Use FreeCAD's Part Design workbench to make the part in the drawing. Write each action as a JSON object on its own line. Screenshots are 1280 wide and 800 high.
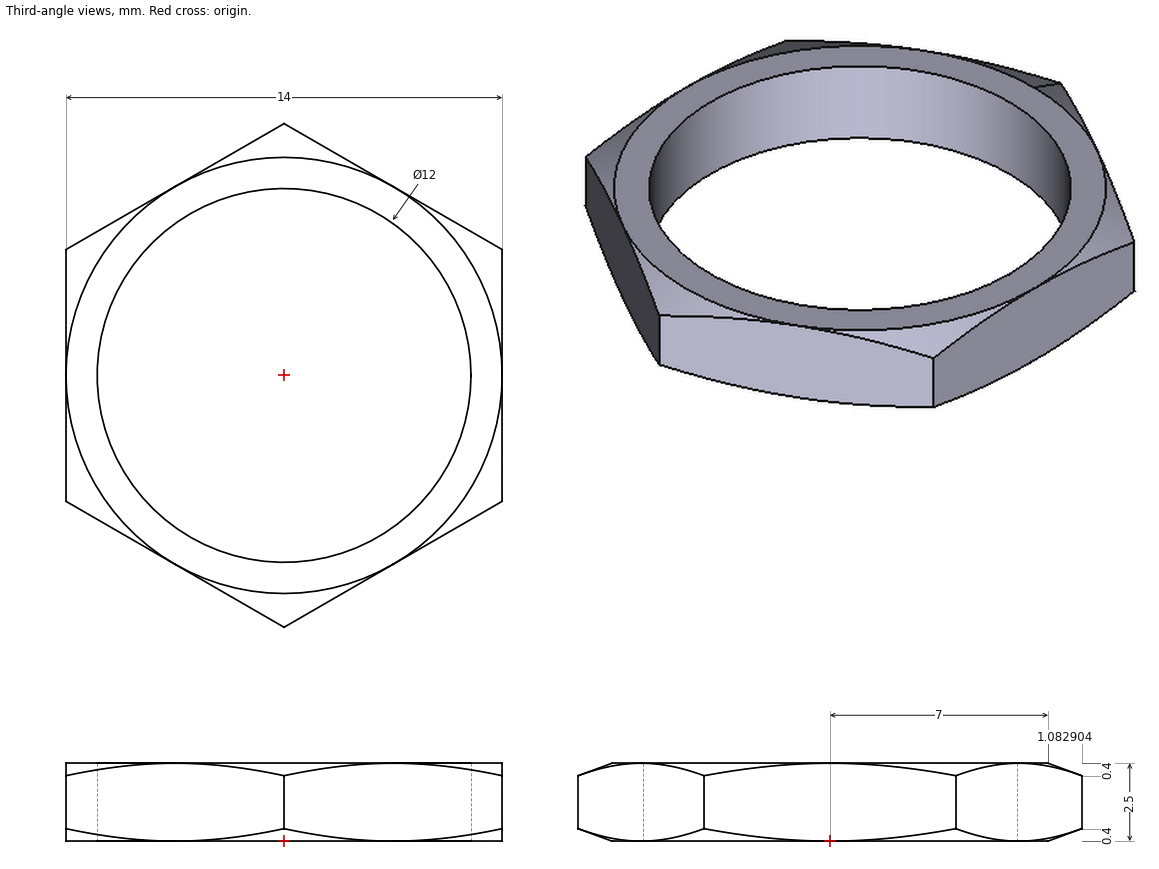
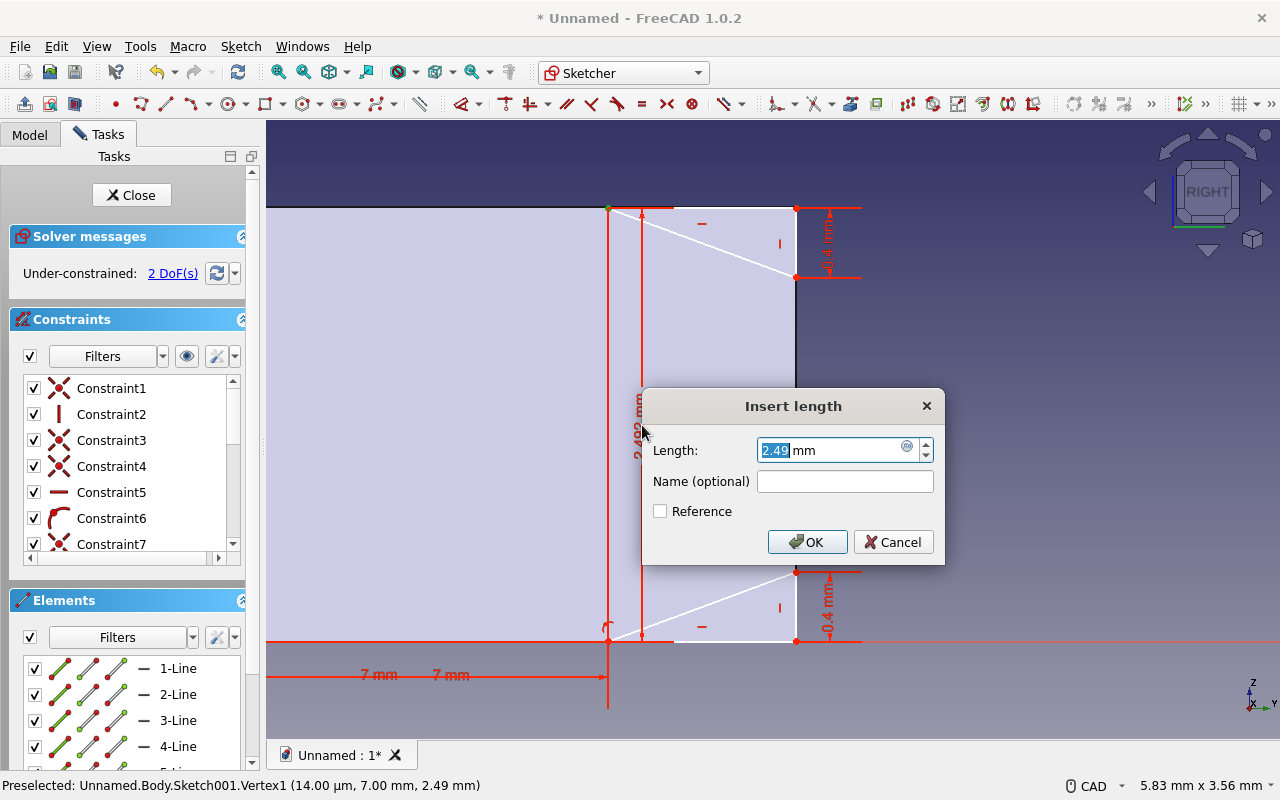
{"action": "type", "text": "2.5"}
{"action": "key", "text": "Return"}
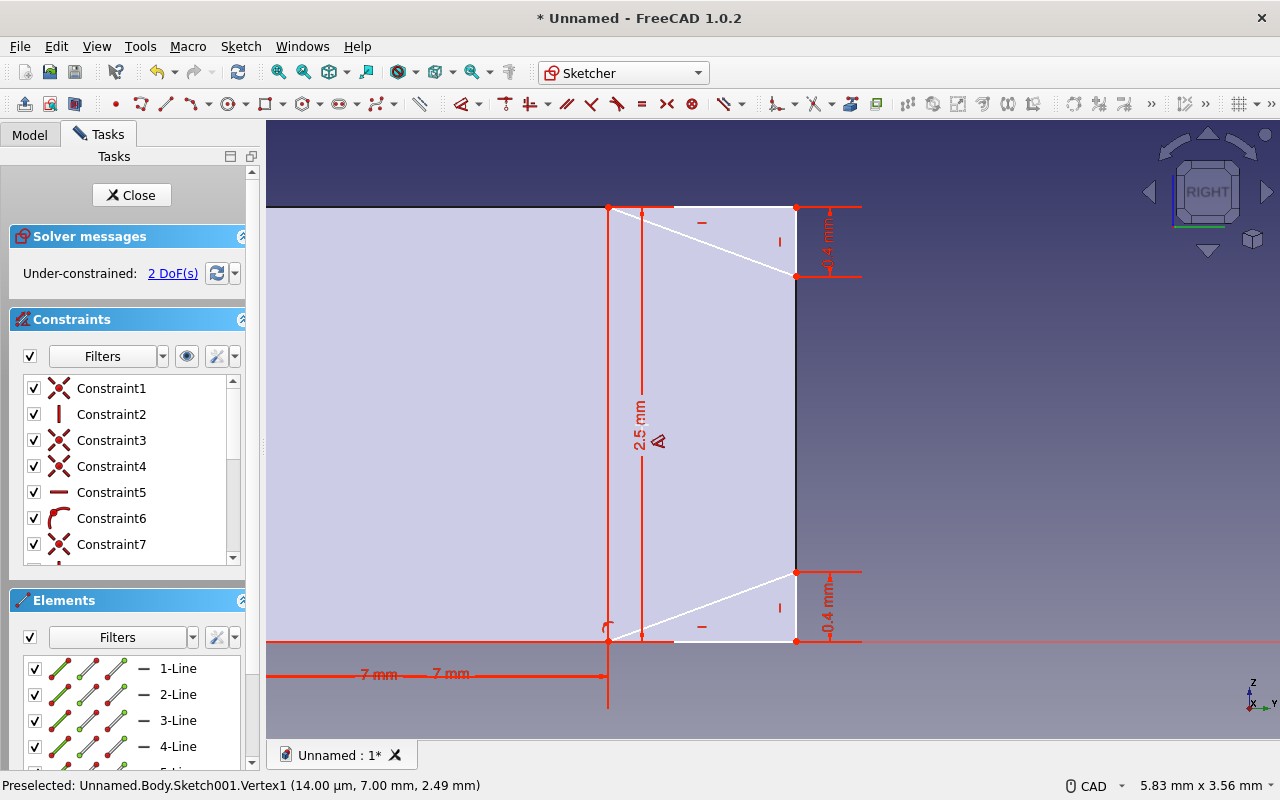
{"action": "left_click", "coordinate": [740, 207]}
{"action": "left_click", "coordinate": [702, 173]}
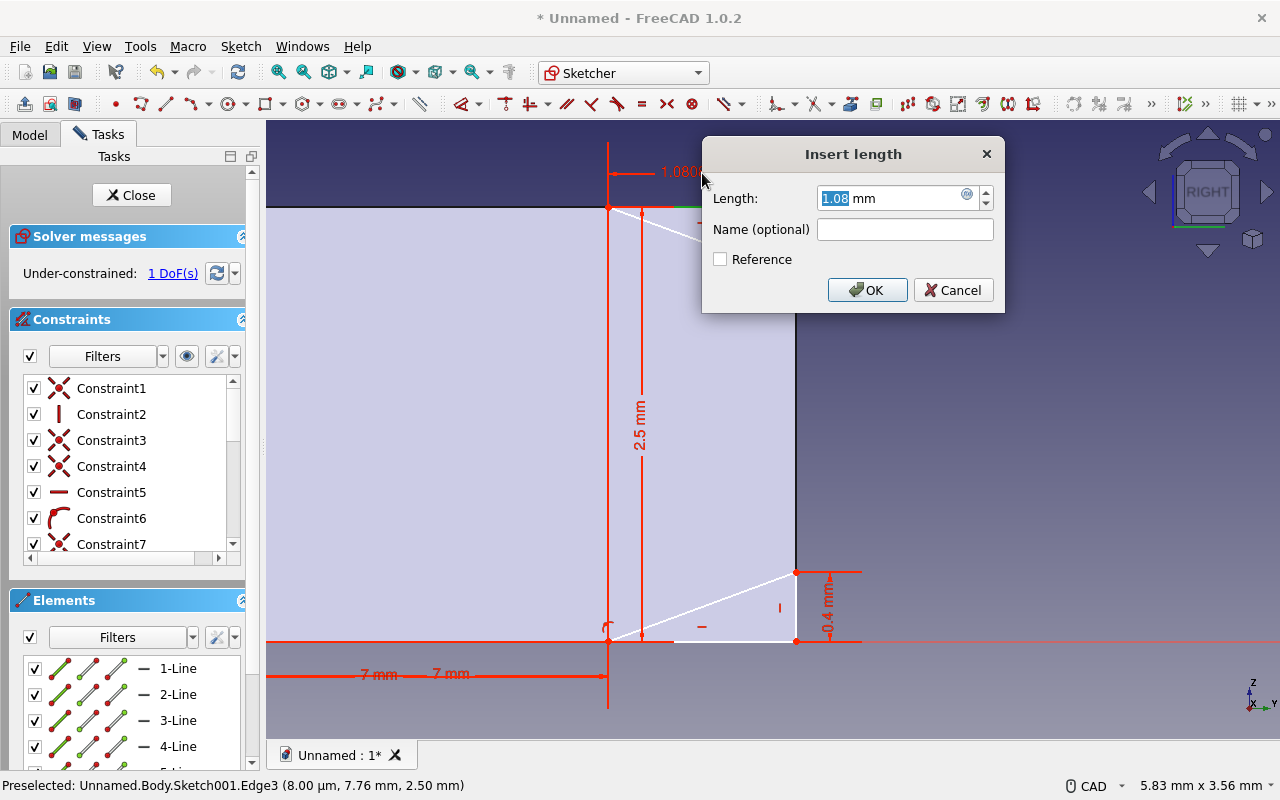
{"action": "type", "text": "1.082904"}
{"action": "key", "text": "Return"}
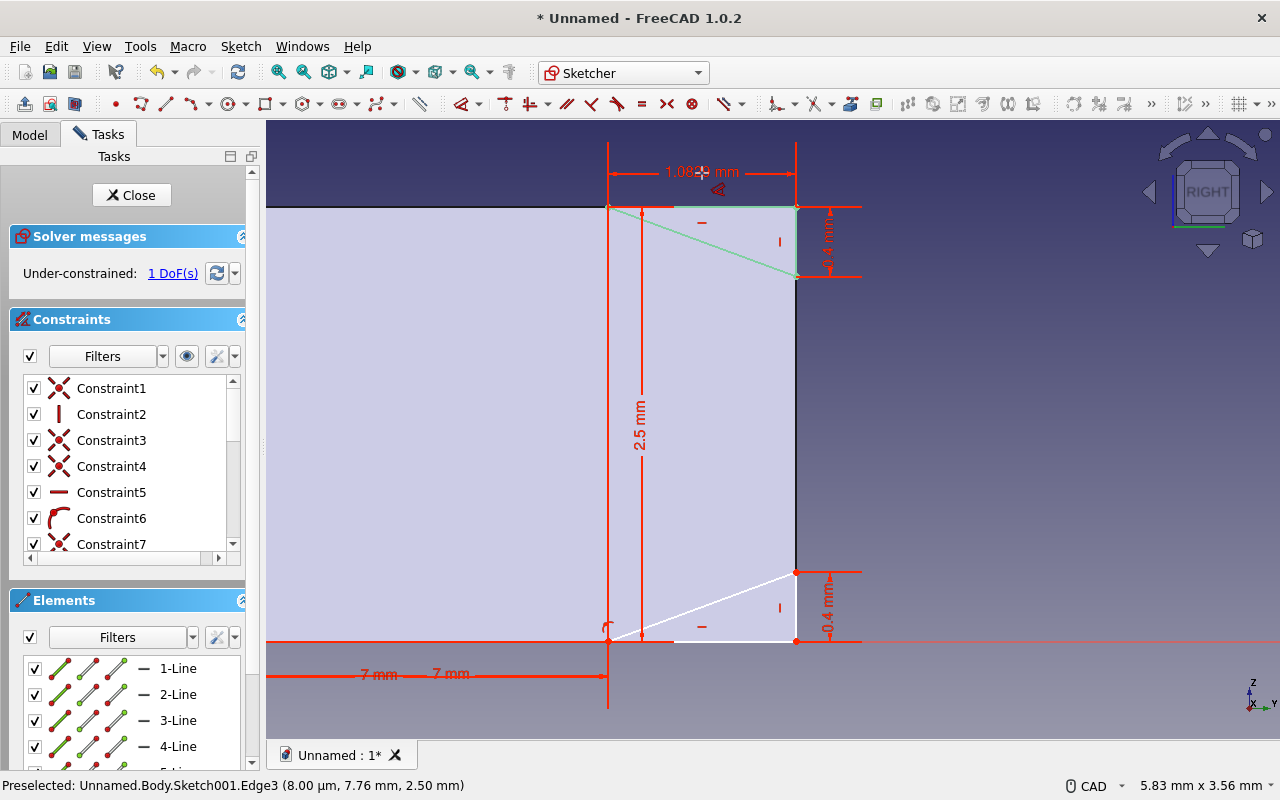
{"action": "left_click", "coordinate": [664, 642]}
{"action": "left_click", "coordinate": [702, 676]}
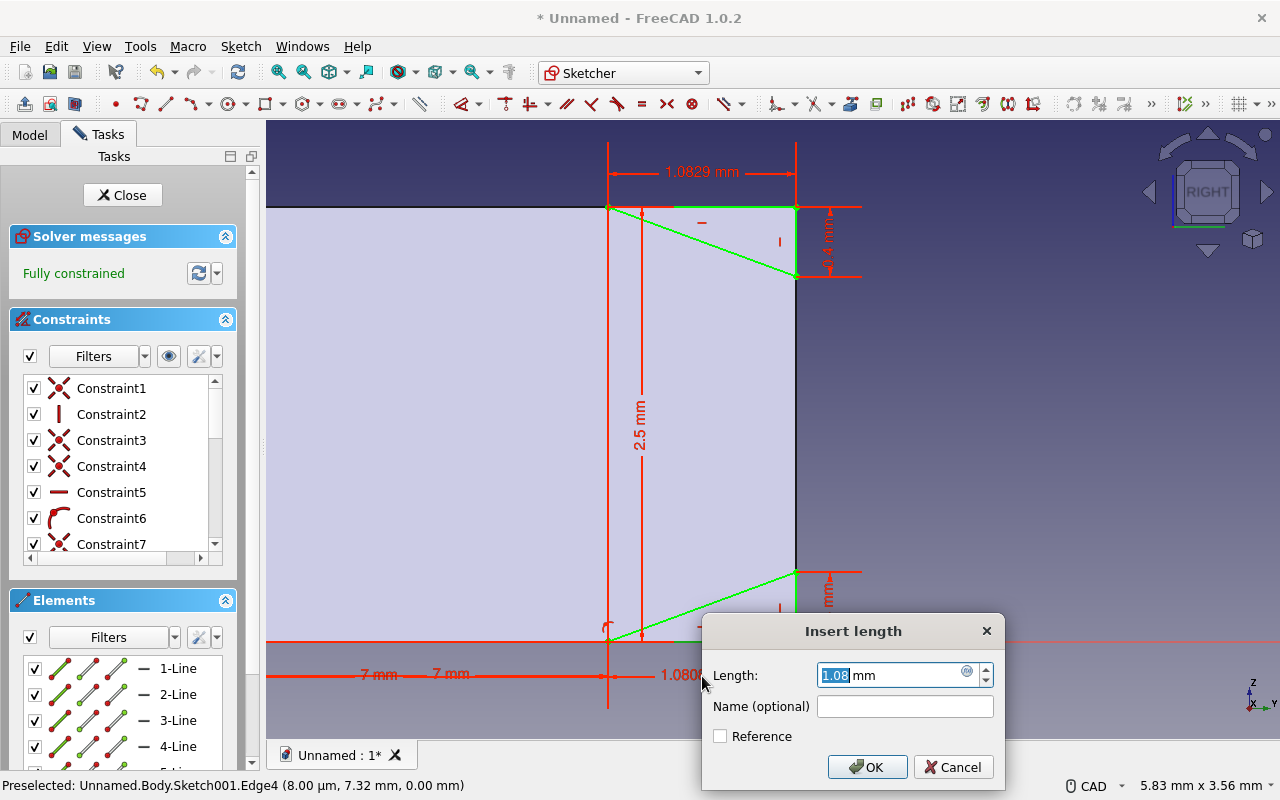
{"action": "type", "text": "1.082904"}
{"action": "key", "text": "Return"}
{"action": "key", "text": "Escape"}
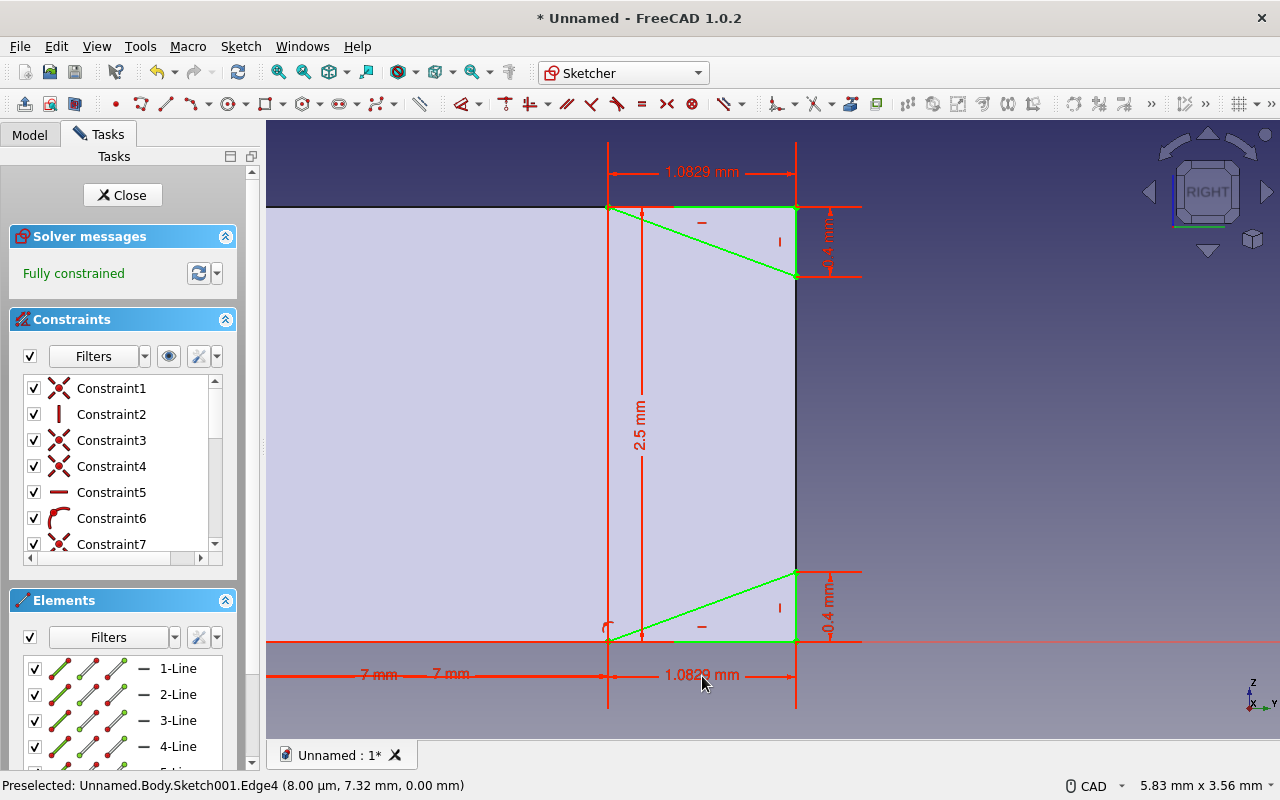
{"action": "left_click", "coordinate": [123, 195]}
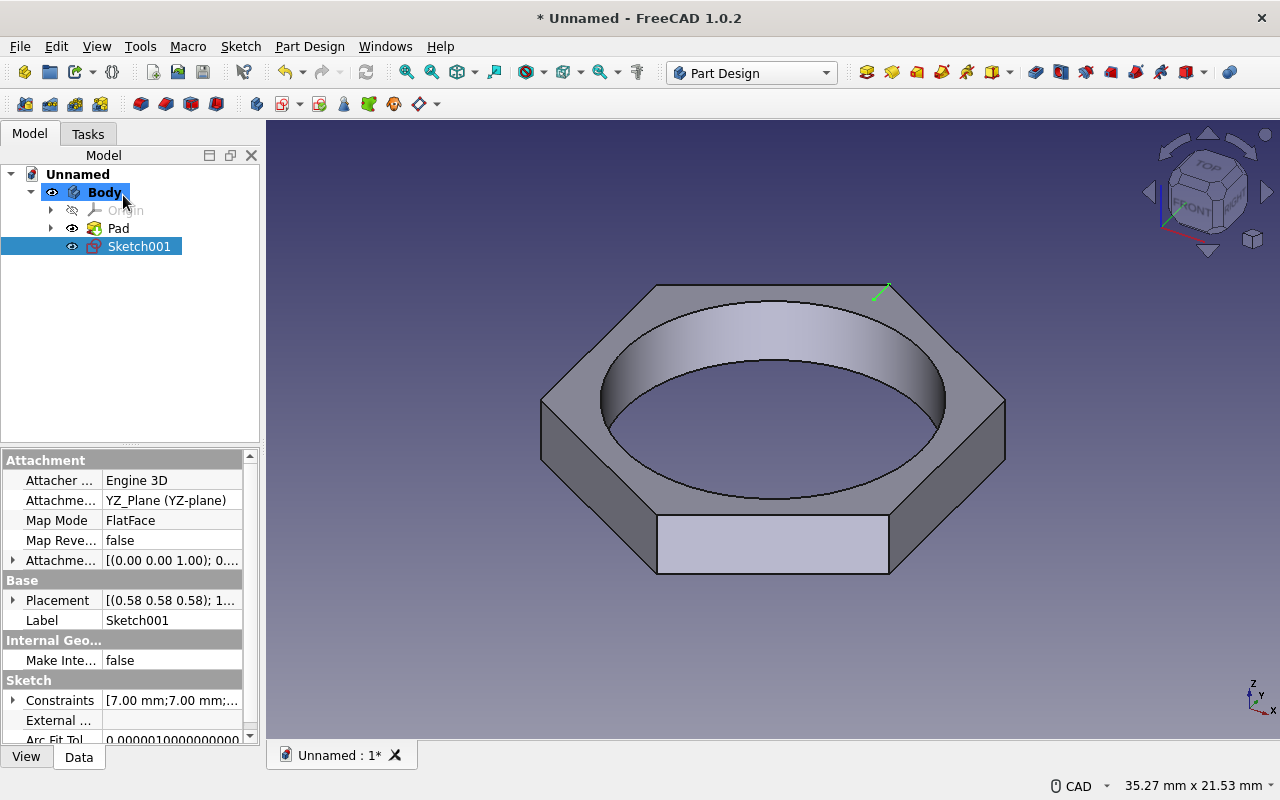
{"action": "left_click", "coordinate": [1086, 72]}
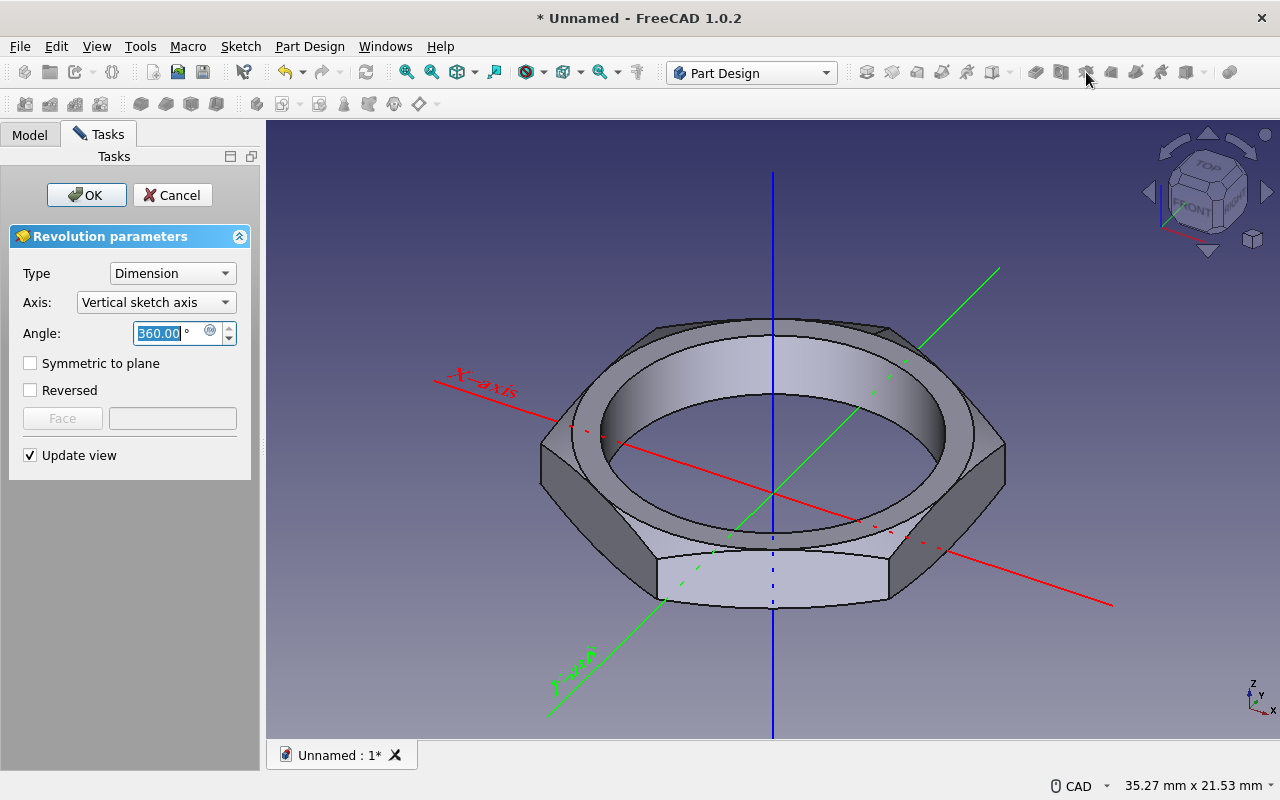
{"action": "left_click", "coordinate": [87, 195]}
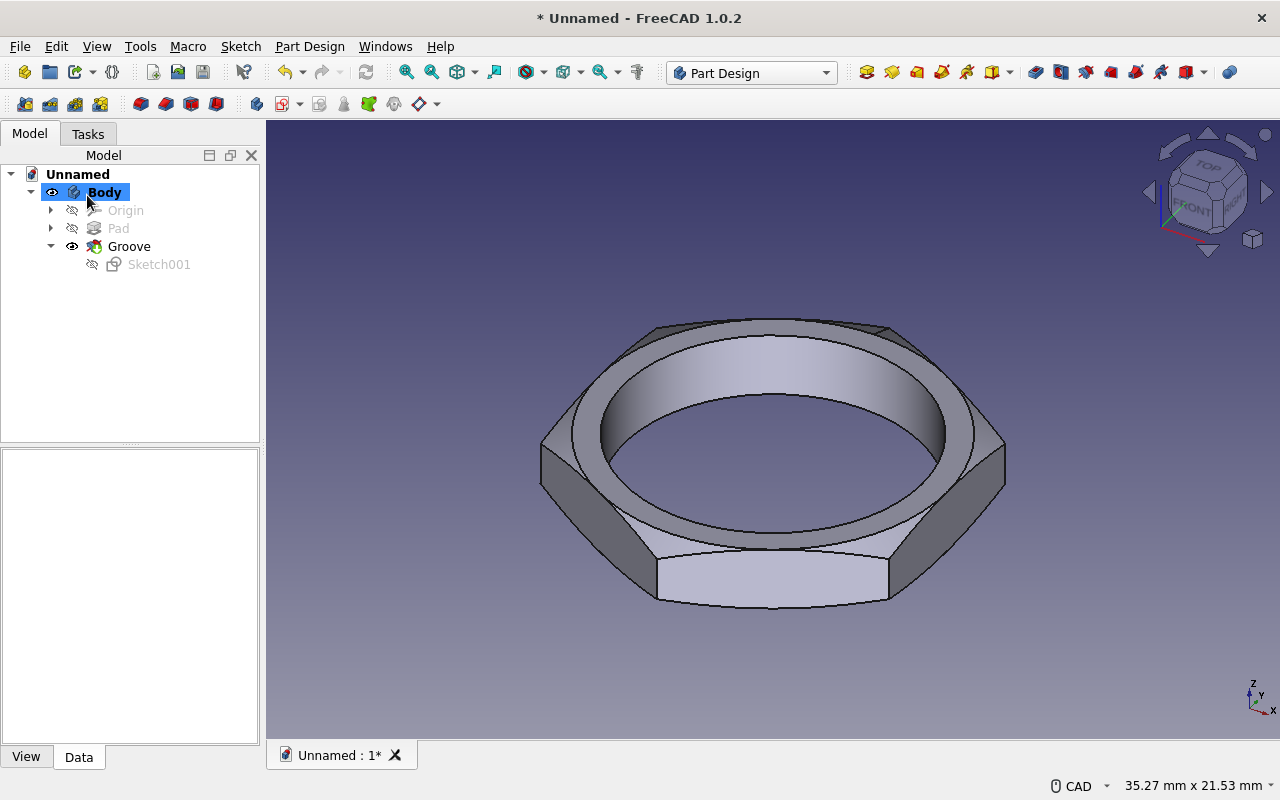
{"action": "key", "text": "0"}